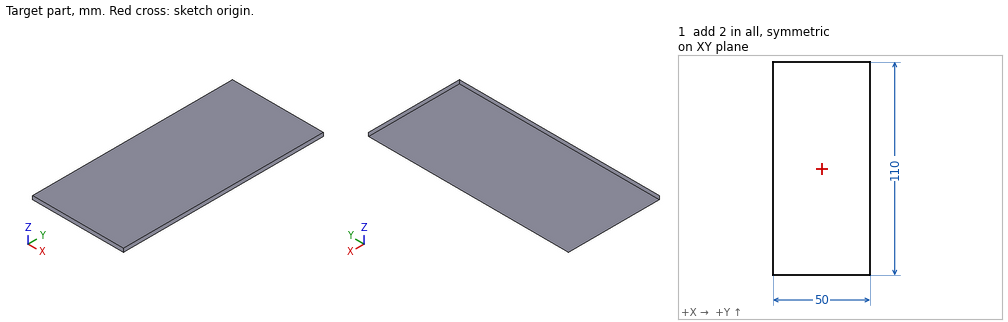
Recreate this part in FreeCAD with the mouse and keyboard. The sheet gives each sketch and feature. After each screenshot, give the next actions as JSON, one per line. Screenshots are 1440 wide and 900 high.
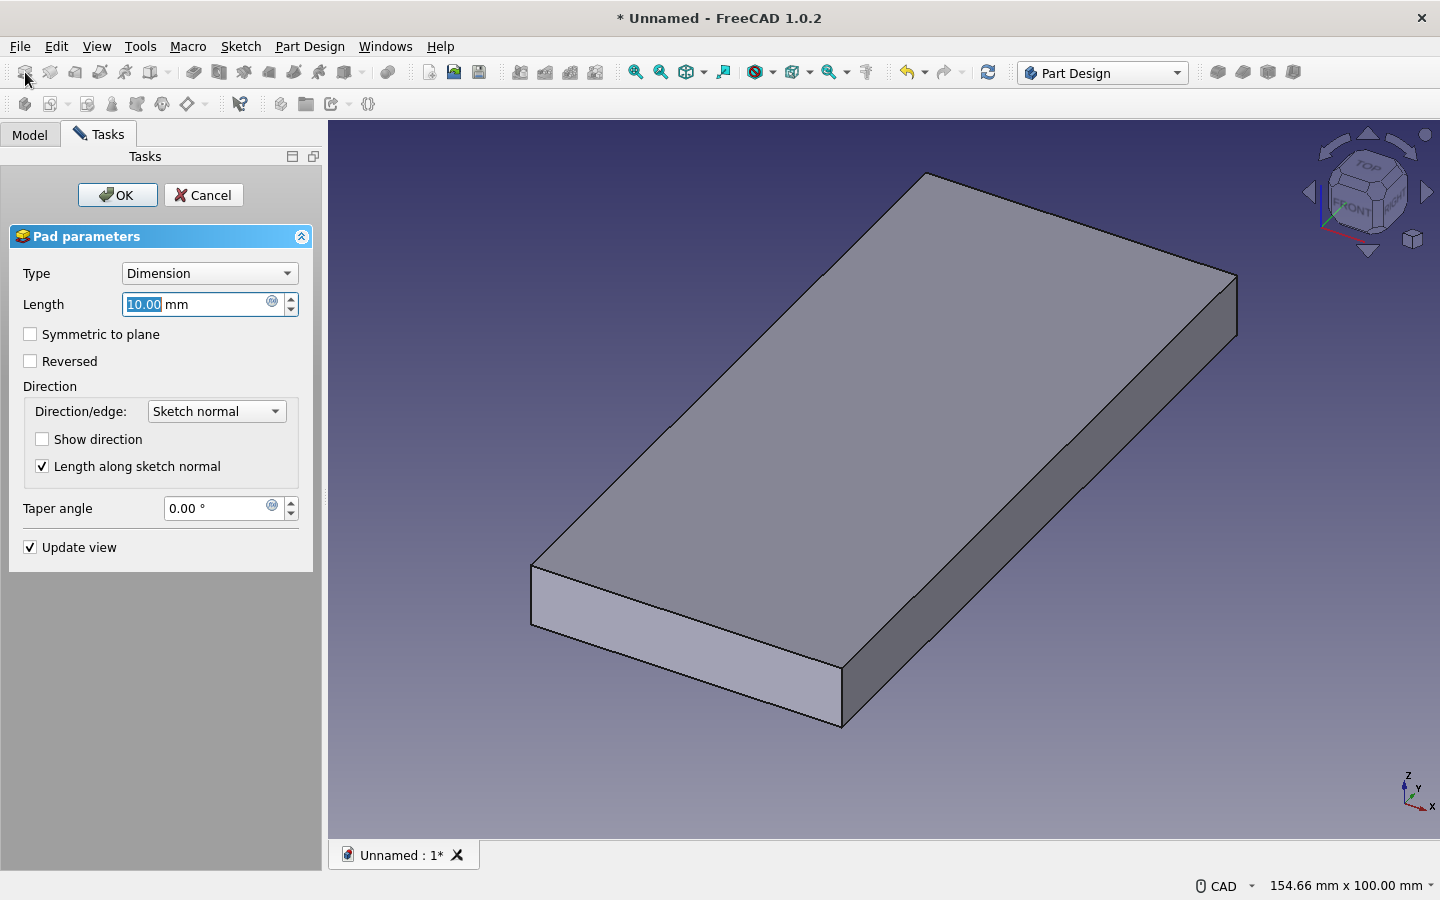
{"action": "type", "text": "2"}
{"action": "key", "text": "Tab"}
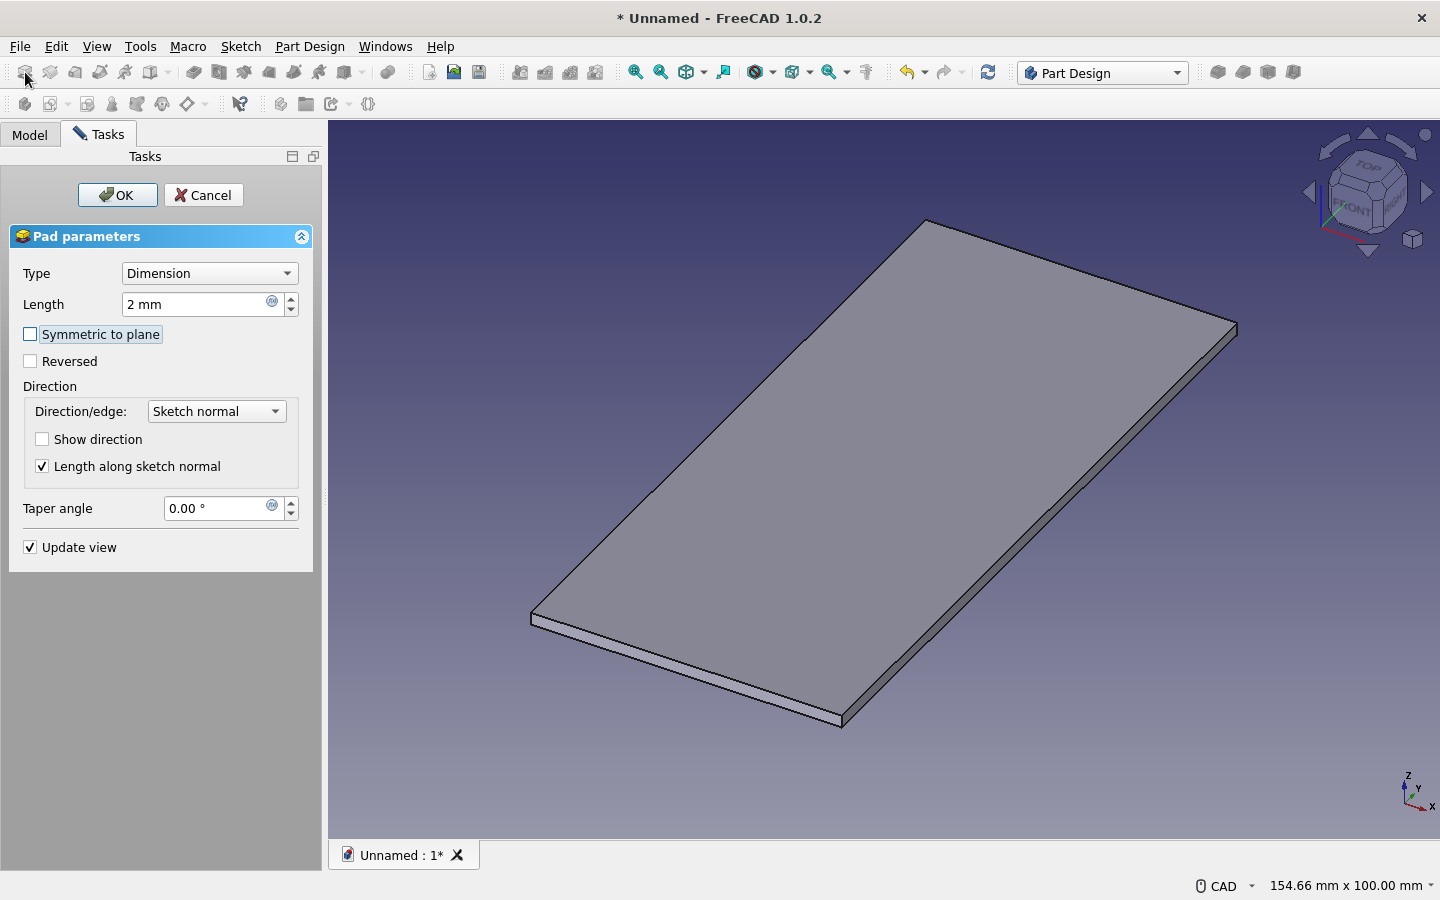
{"action": "left_click", "coordinate": [31, 334]}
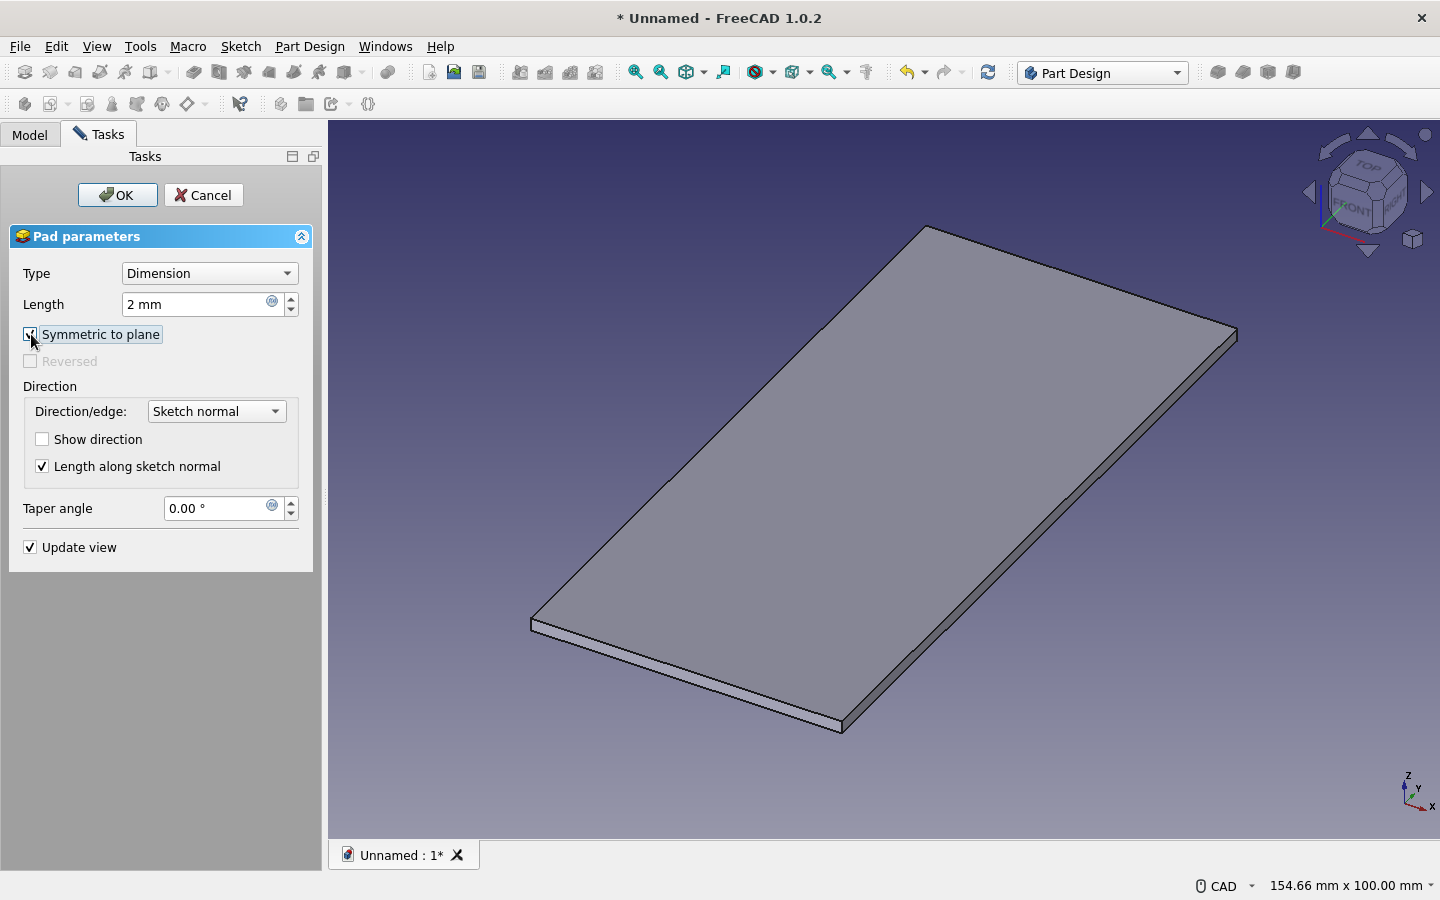
{"action": "left_click", "coordinate": [118, 195]}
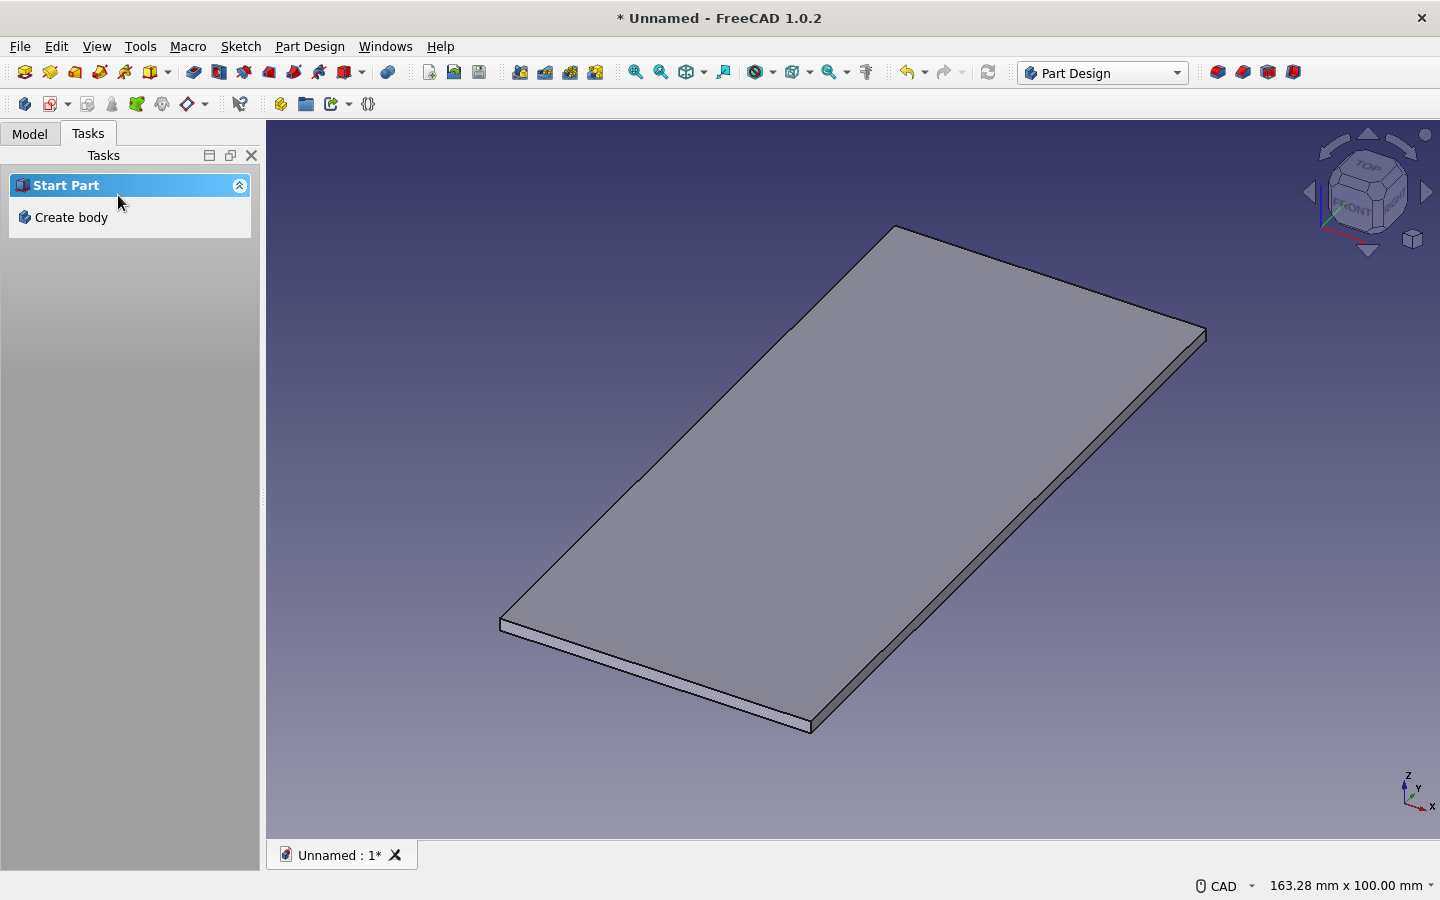
{"action": "key", "text": "0"}